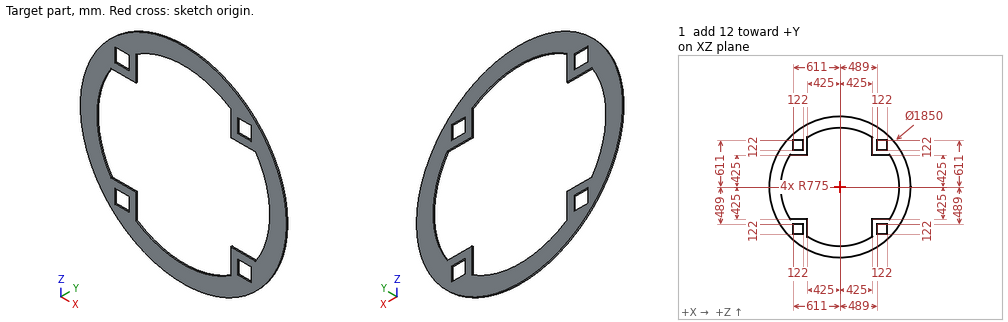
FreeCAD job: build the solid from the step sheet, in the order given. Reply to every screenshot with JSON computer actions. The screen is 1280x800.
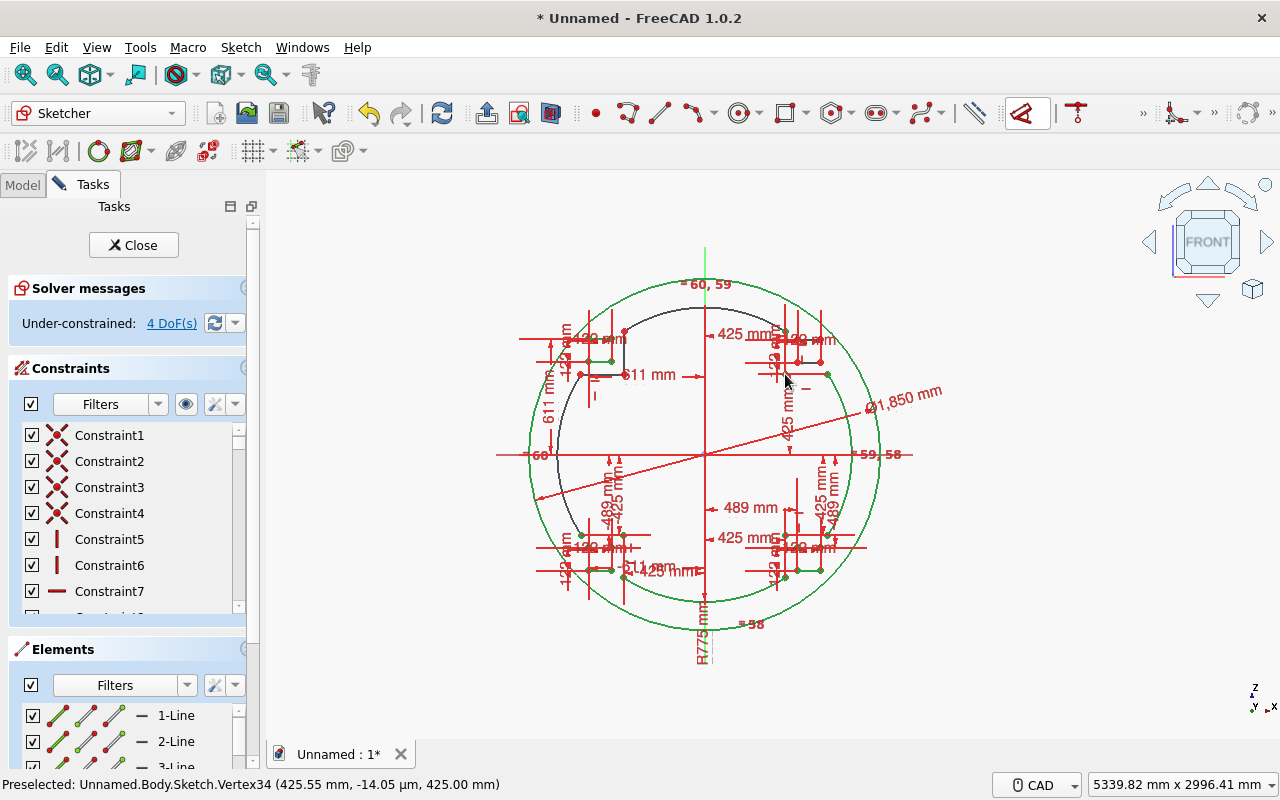
{"action": "left_click", "coordinate": [624, 332]}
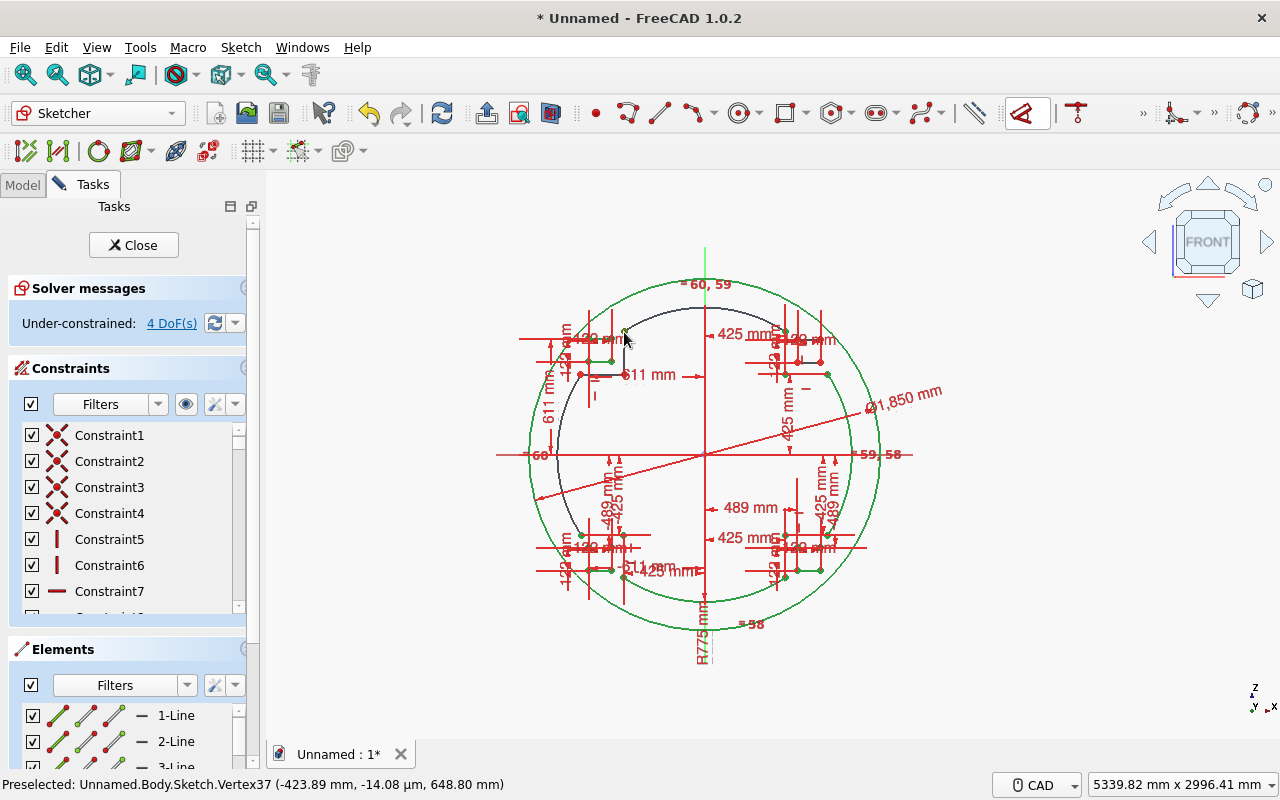
{"action": "key", "text": "l"}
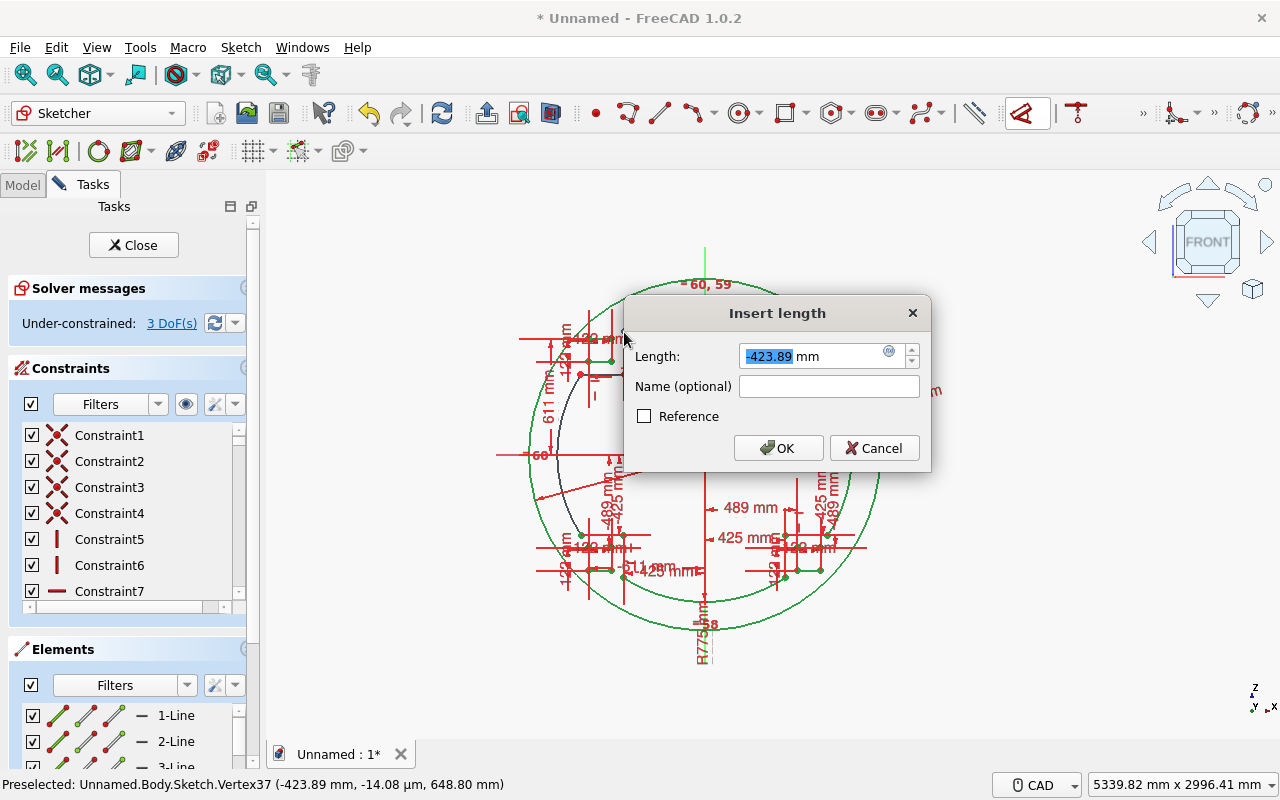
{"action": "type", "text": "-425"}
{"action": "key", "text": "Return"}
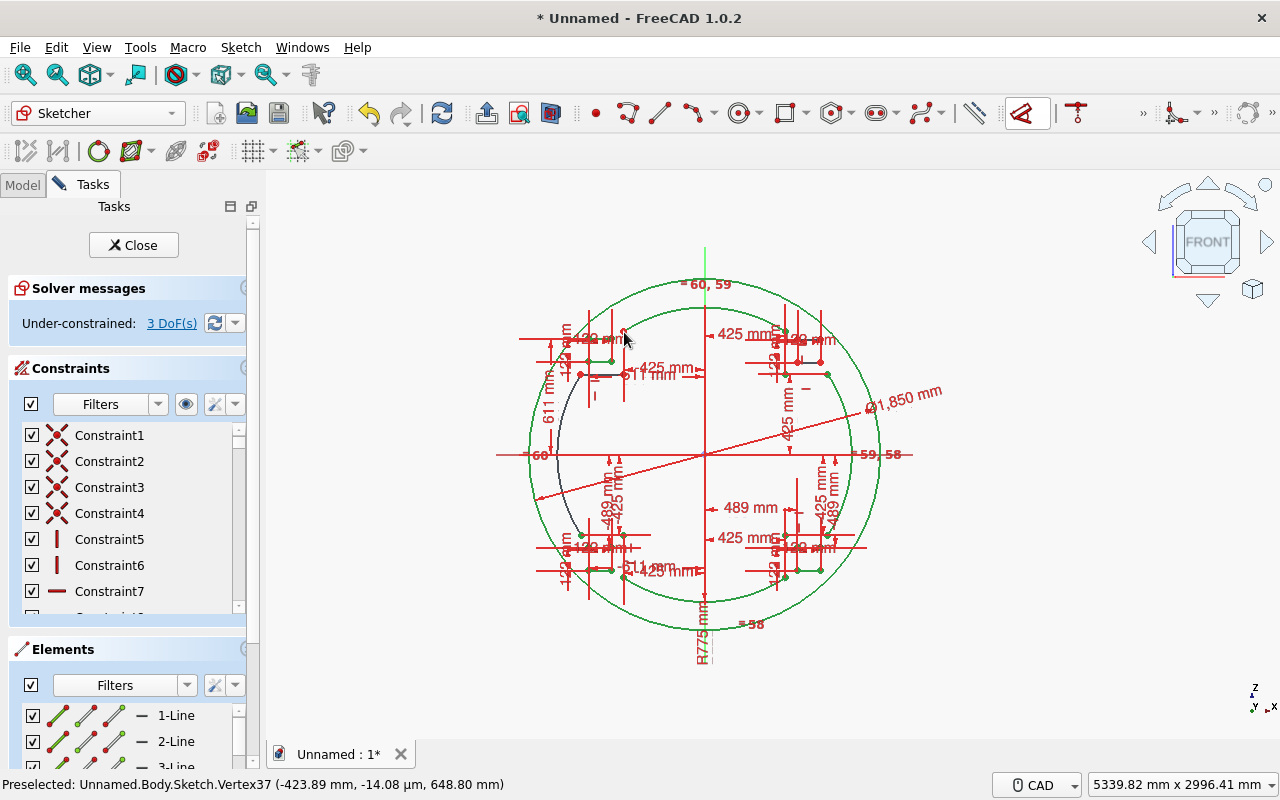
{"action": "left_click", "coordinate": [624, 375]}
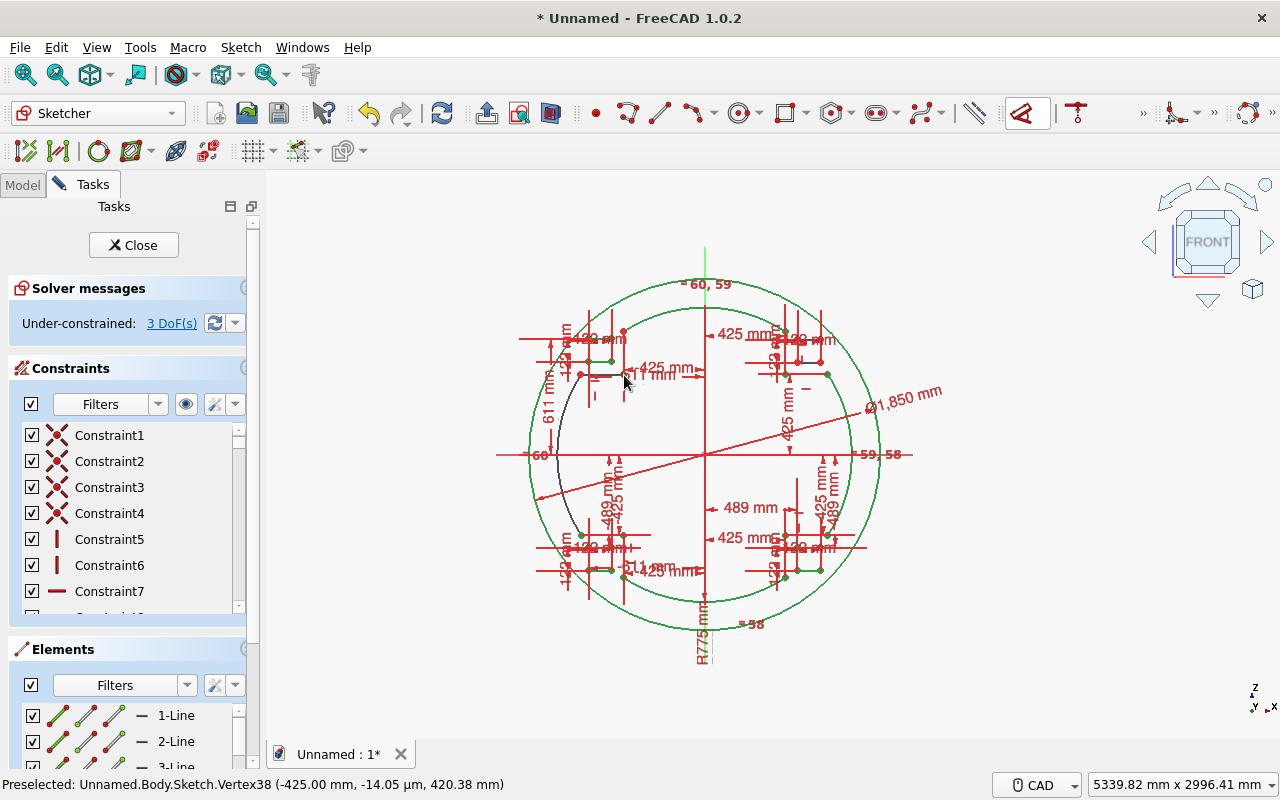
{"action": "key", "text": "i"}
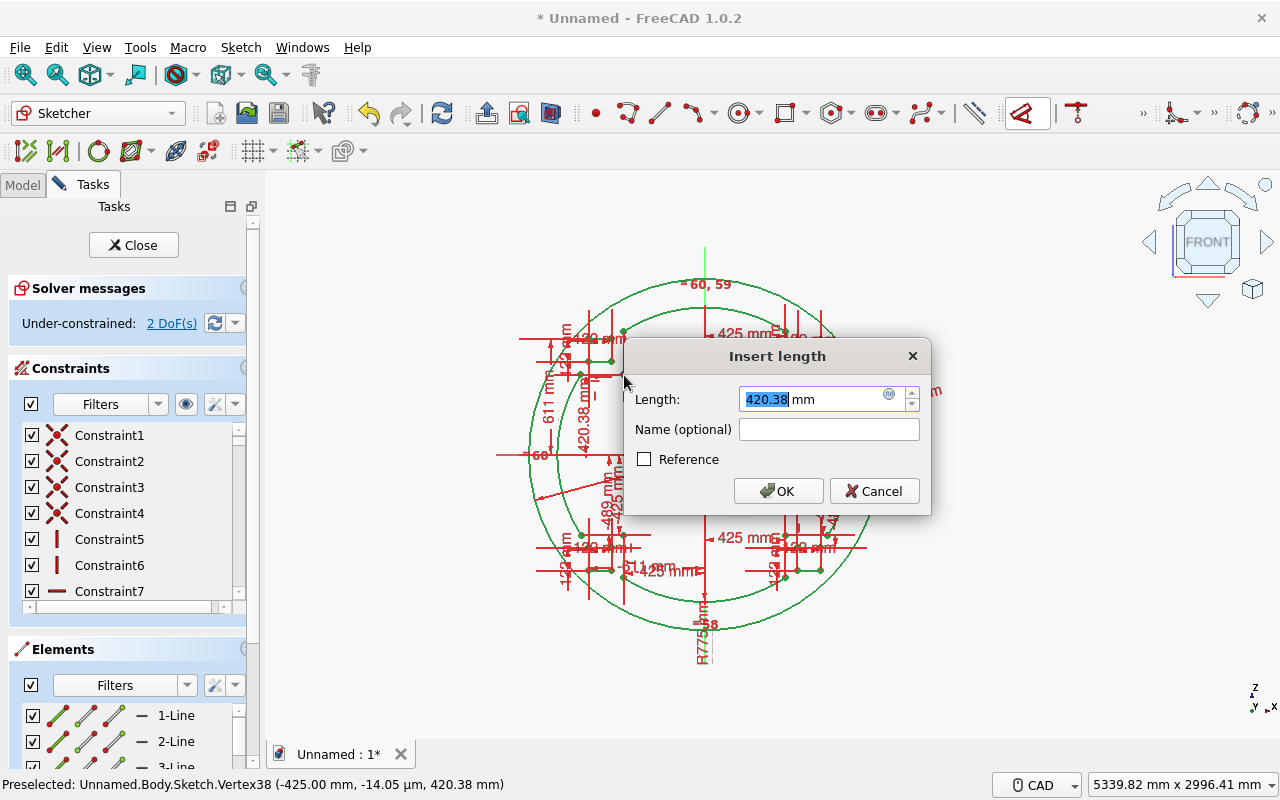
{"action": "type", "text": "425"}
{"action": "key", "text": "Return"}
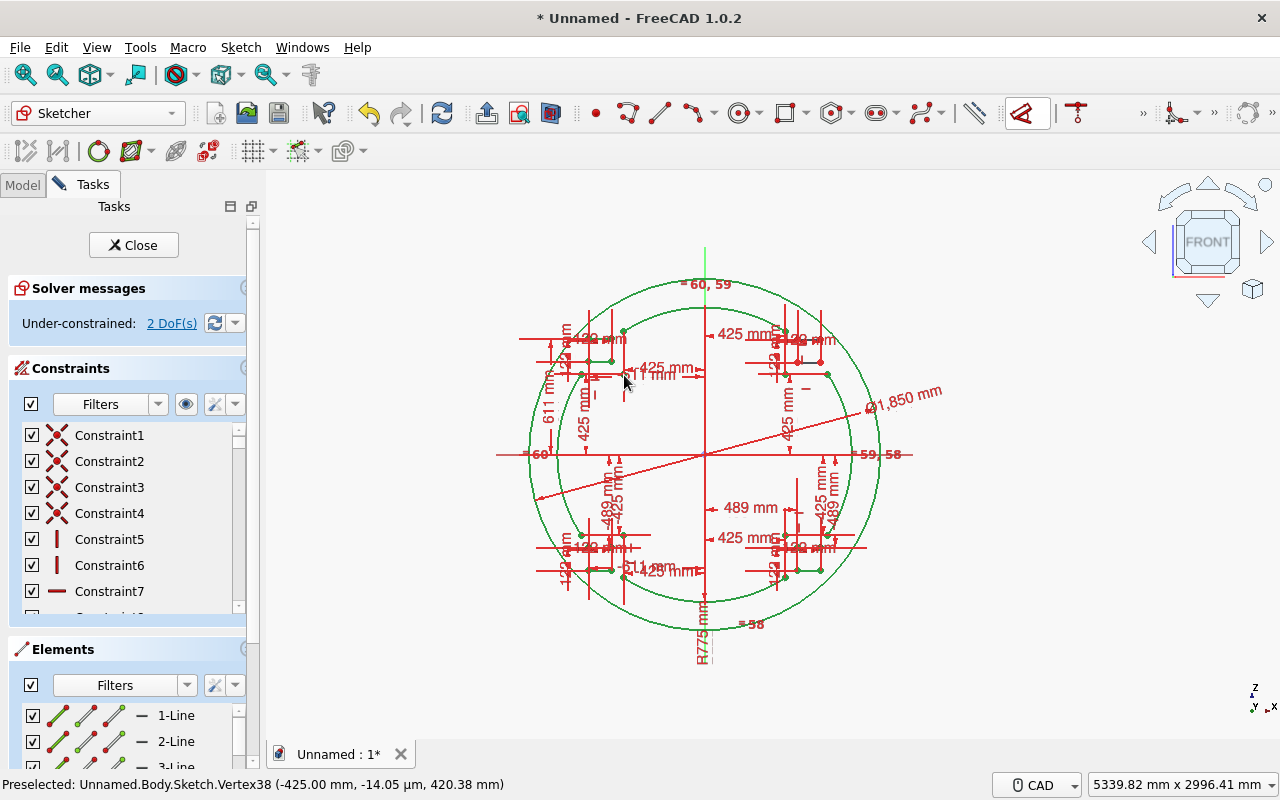
{"action": "left_click", "coordinate": [798, 340]}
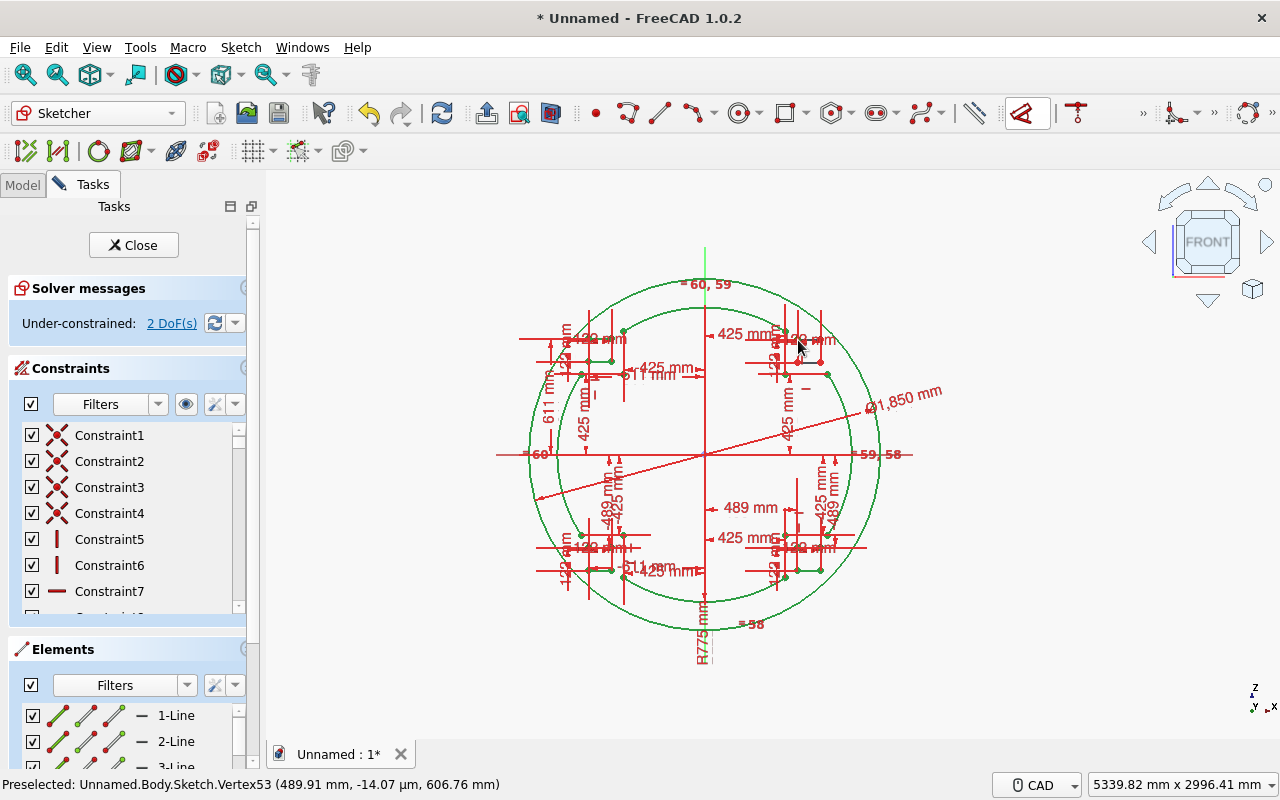
{"action": "key", "text": "l"}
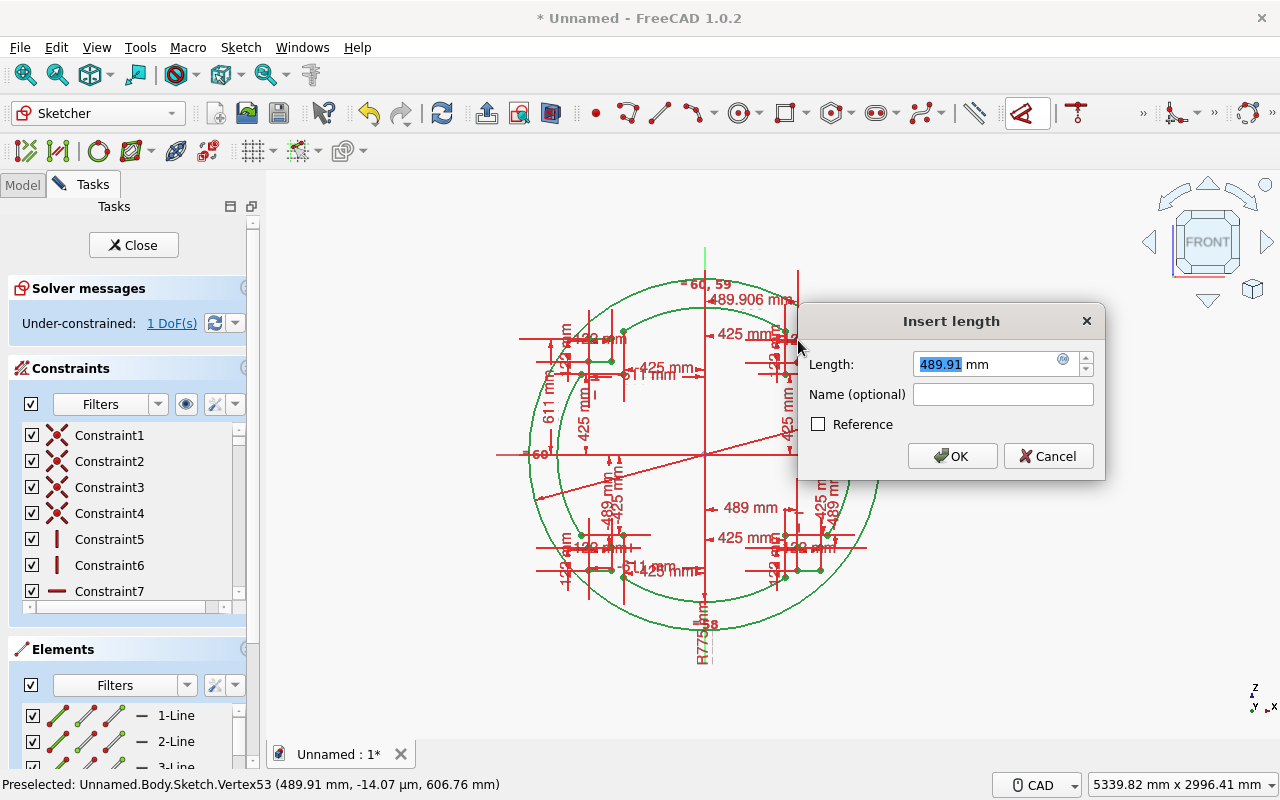
{"action": "type", "text": "489"}
{"action": "key", "text": "Return"}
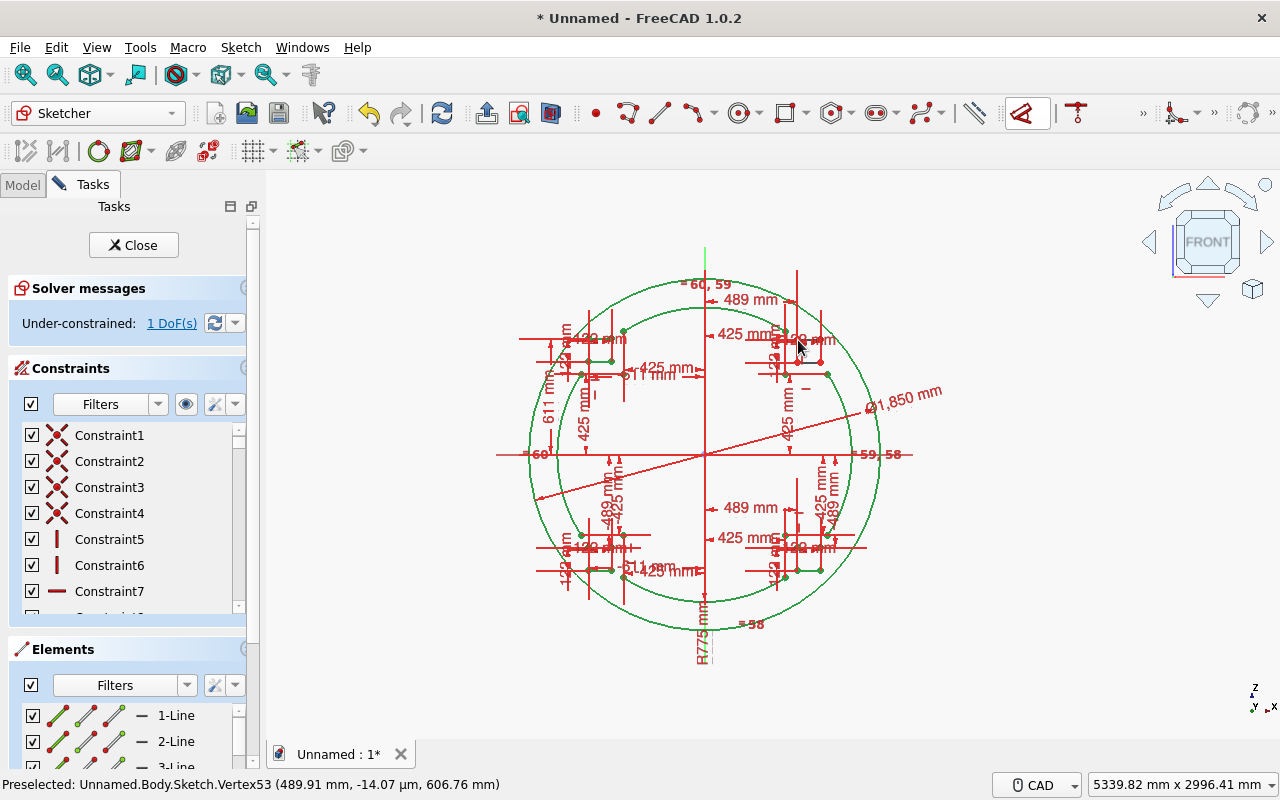
{"action": "left_click", "coordinate": [797, 340]}